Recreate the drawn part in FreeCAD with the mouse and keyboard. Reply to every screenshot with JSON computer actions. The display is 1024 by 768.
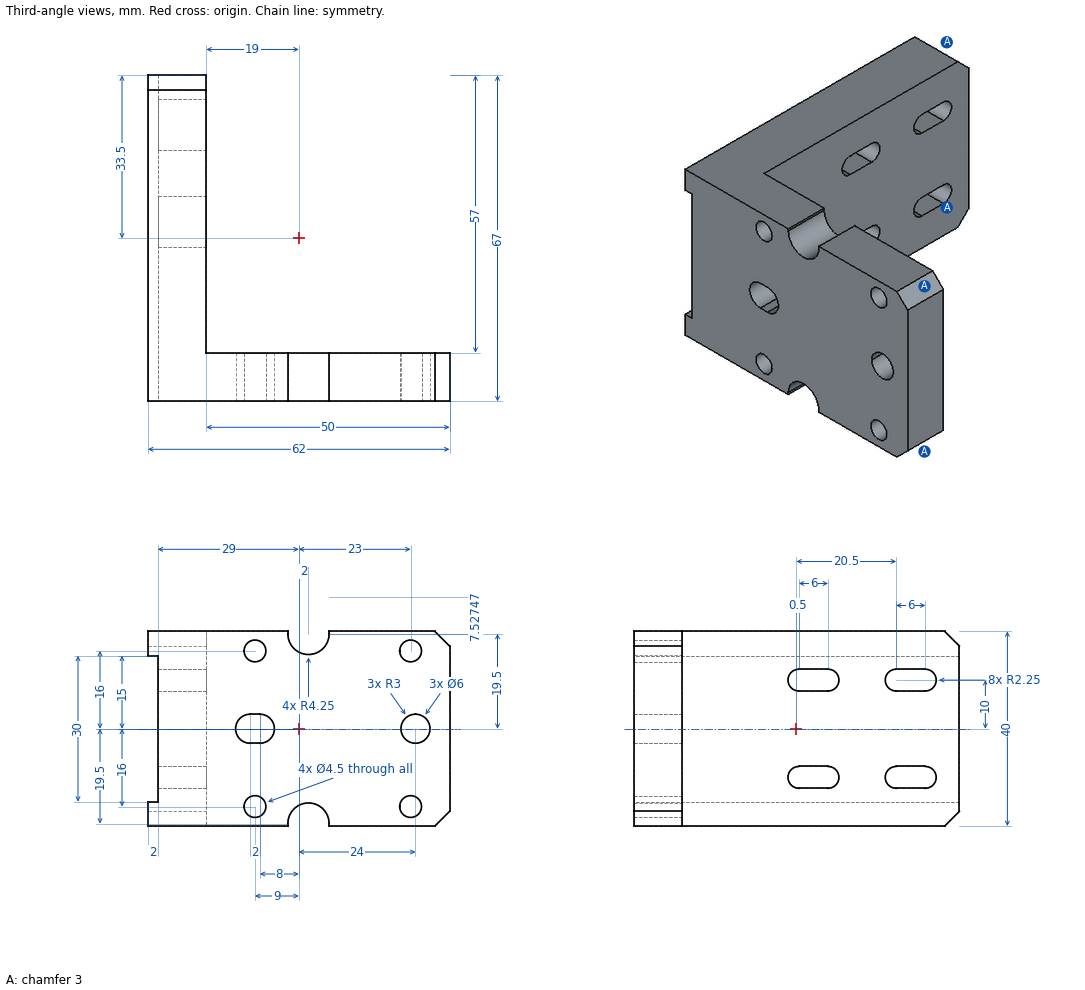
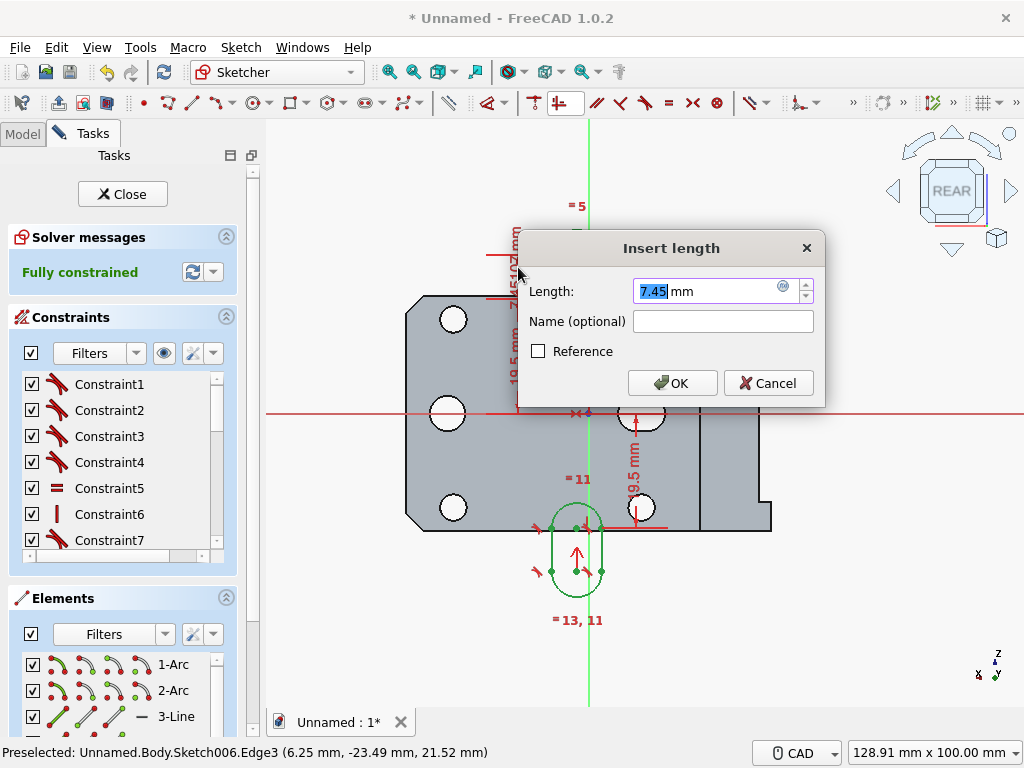
{"action": "type", "text": "7.52747"}
{"action": "key", "text": "Return"}
{"action": "key", "text": "Escape"}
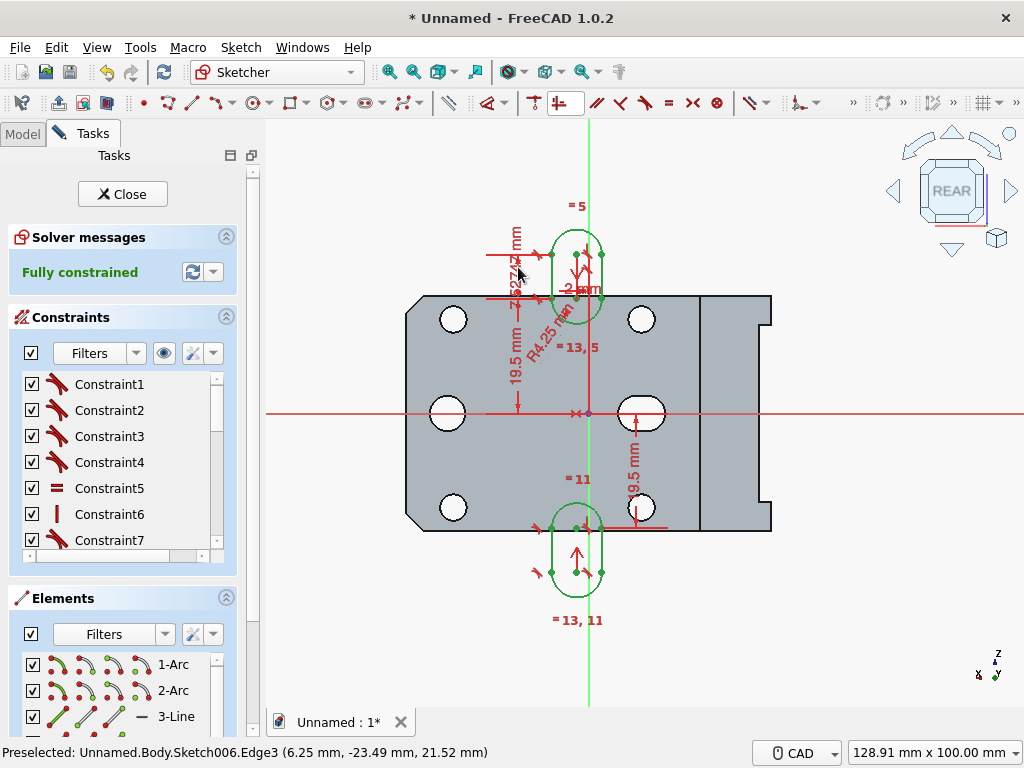
{"action": "left_click", "coordinate": [123, 194]}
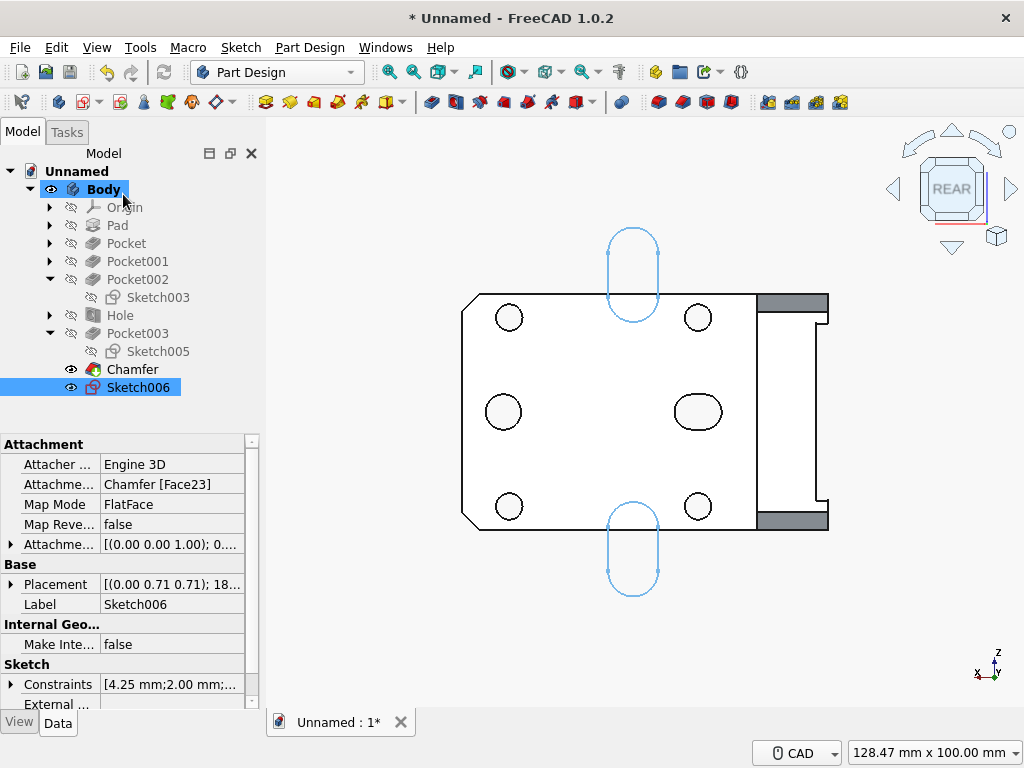
{"action": "left_click", "coordinate": [432, 102]}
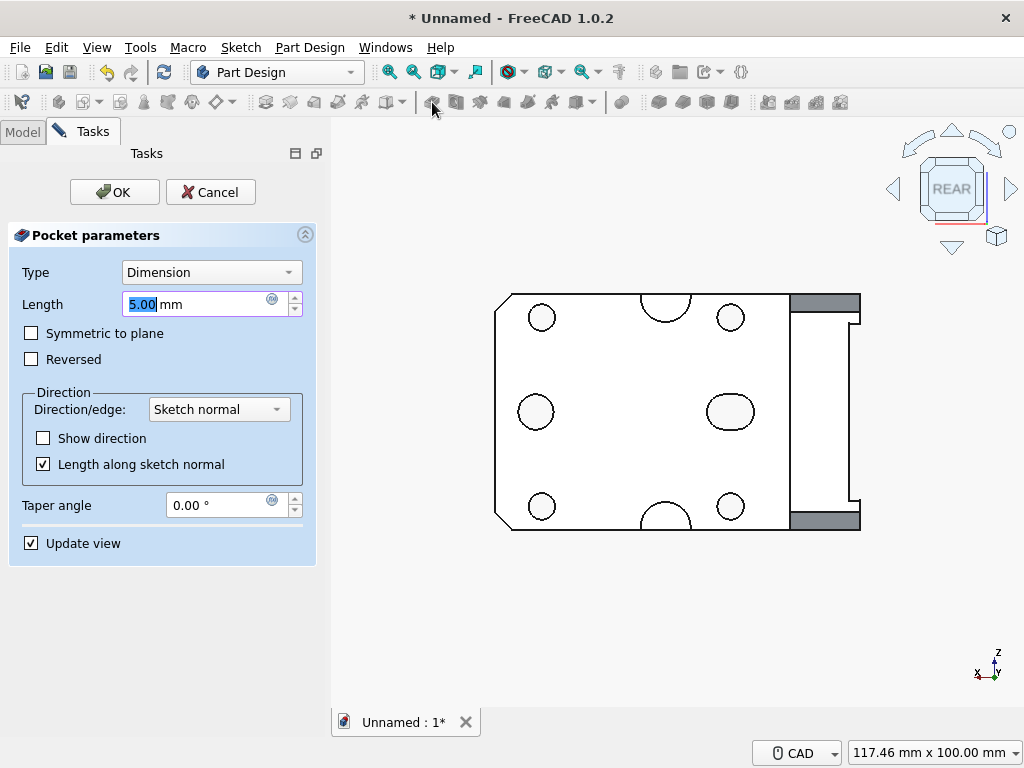
{"action": "left_click", "coordinate": [212, 272]}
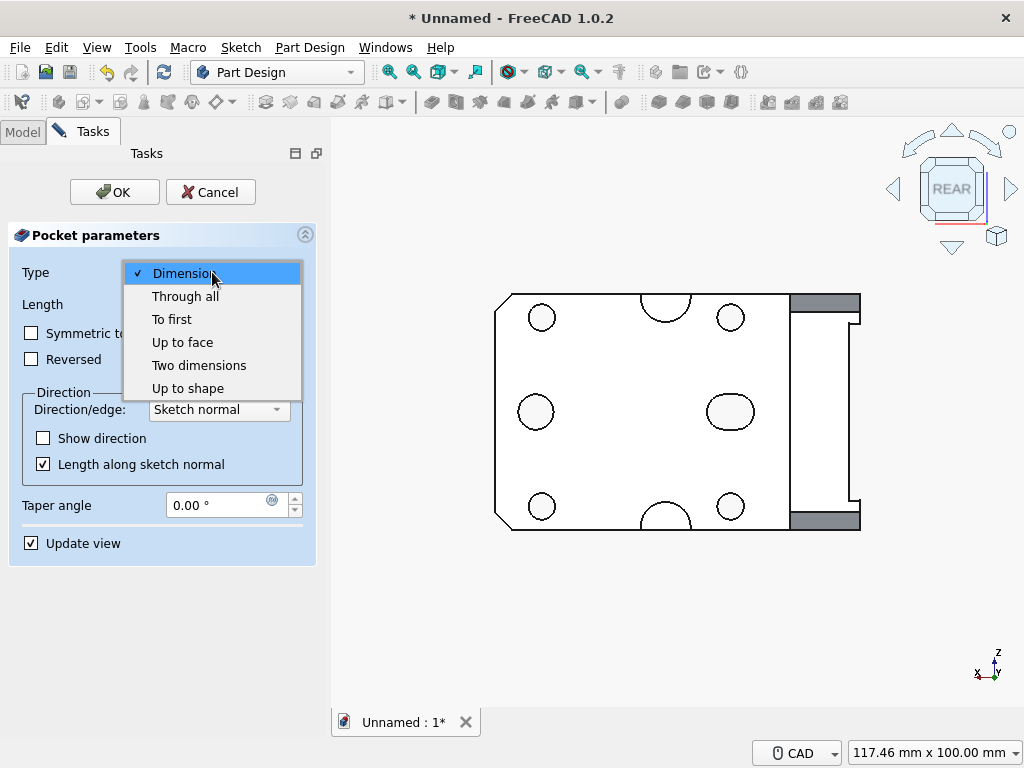
{"action": "left_click", "coordinate": [212, 296]}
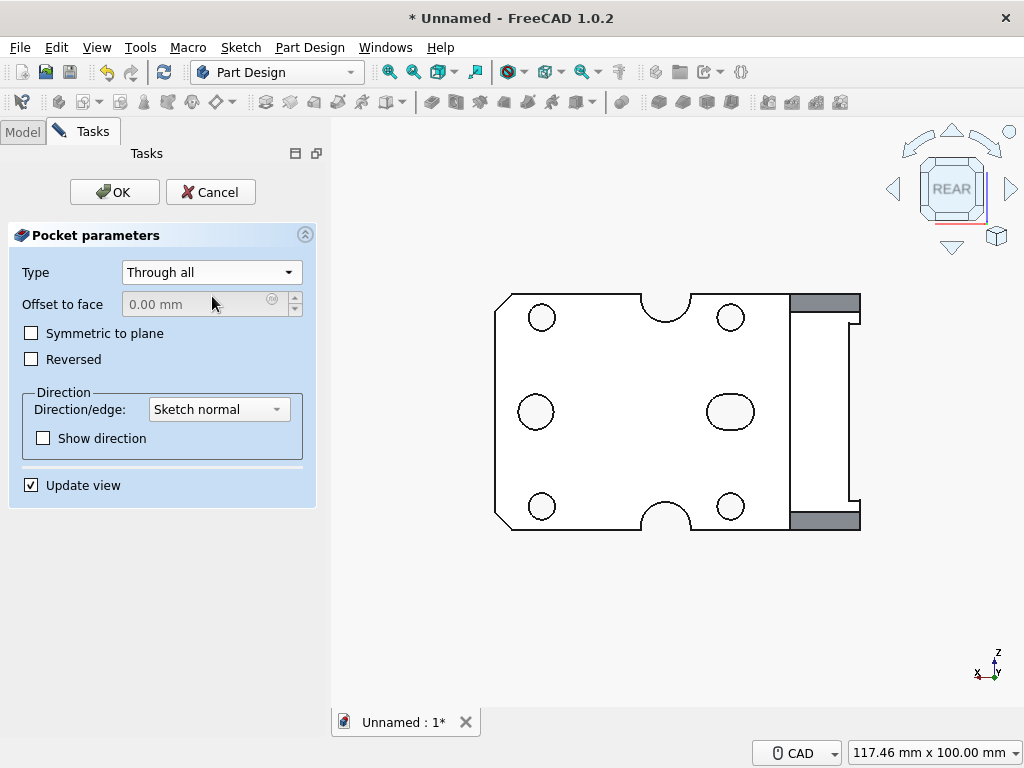
{"action": "left_click", "coordinate": [115, 192]}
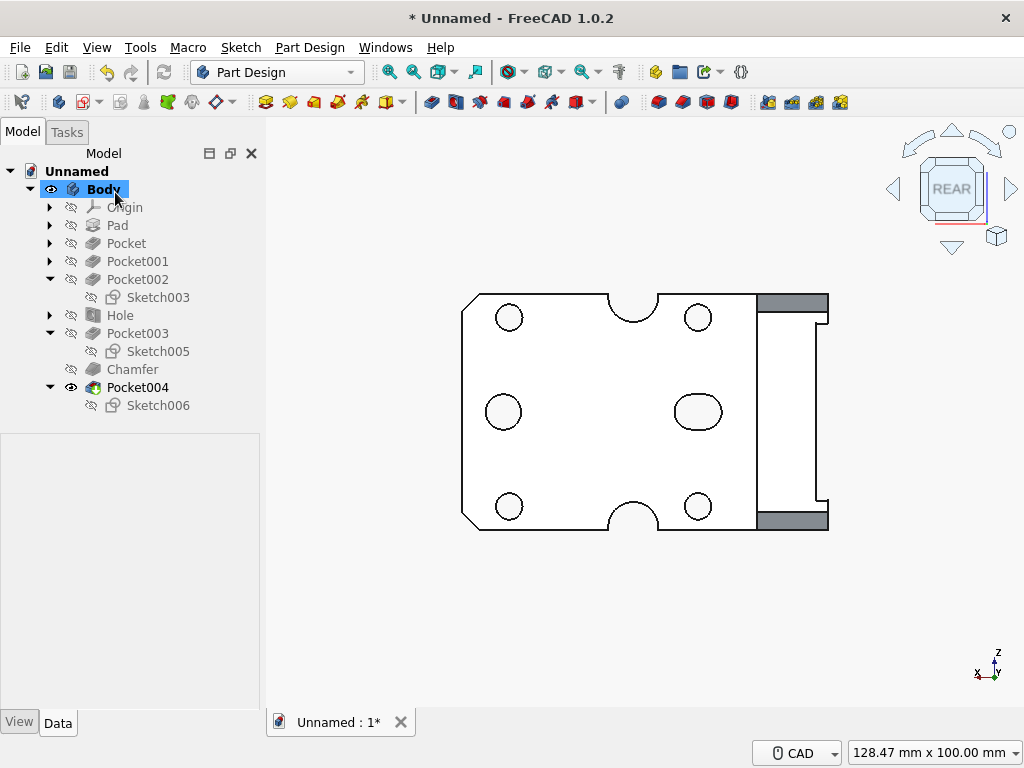
{"action": "key", "text": "0"}